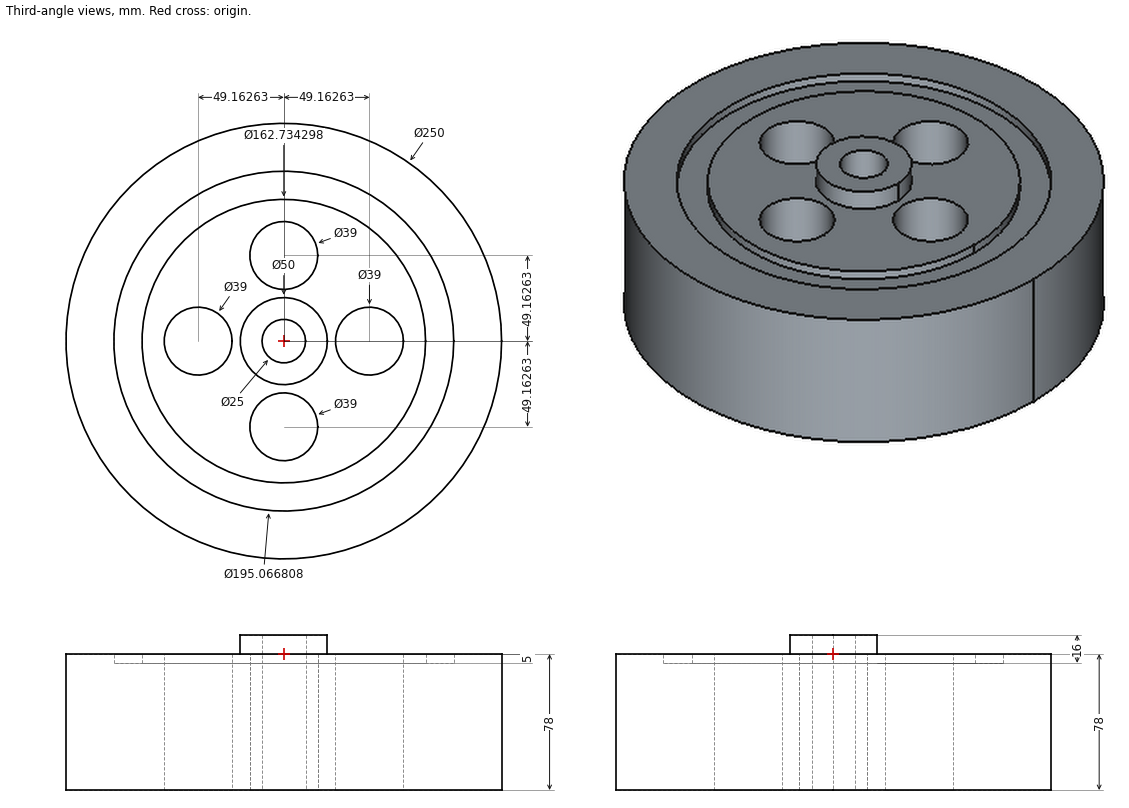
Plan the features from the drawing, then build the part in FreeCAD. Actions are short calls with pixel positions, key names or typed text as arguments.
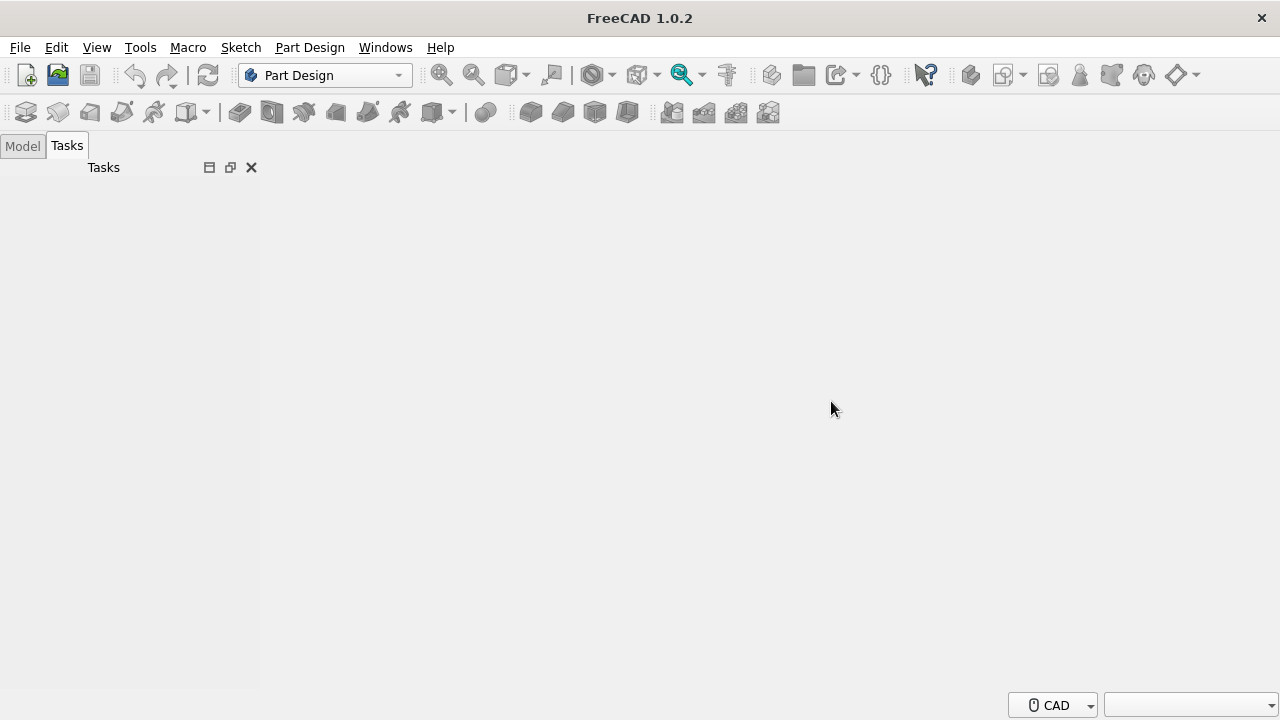
click(26, 76)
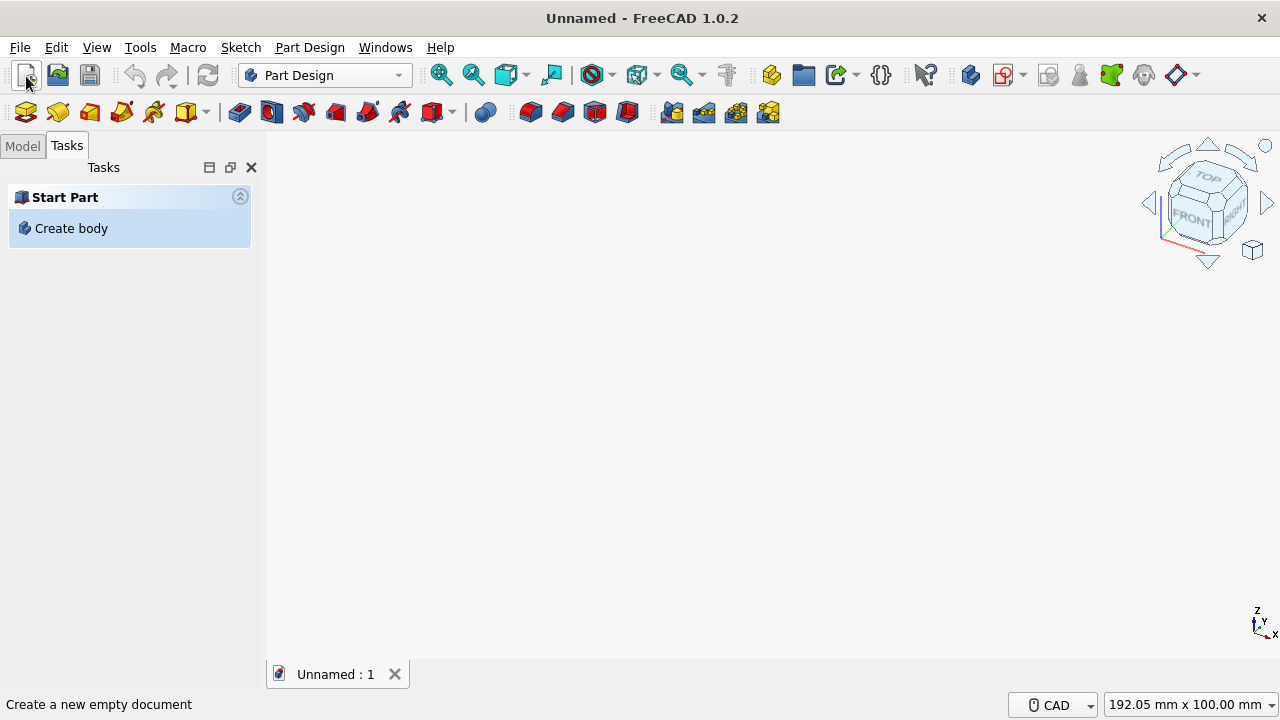
click(1004, 76)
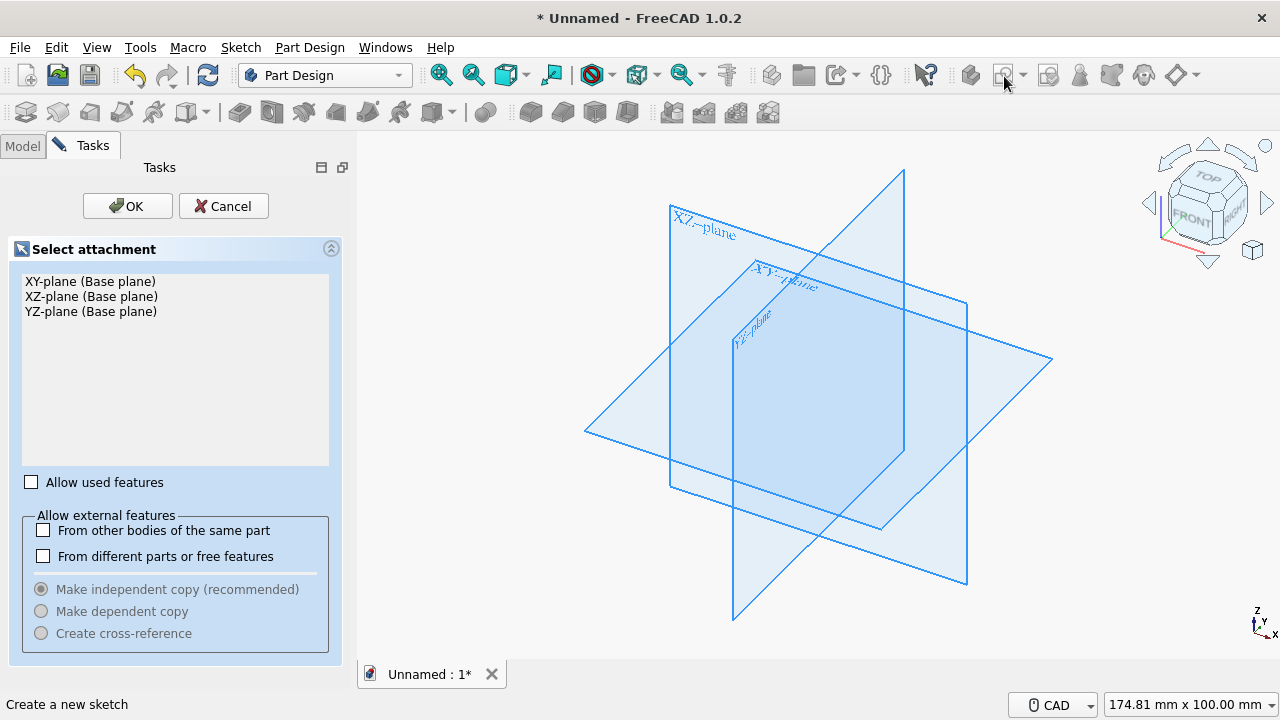
click(82, 282)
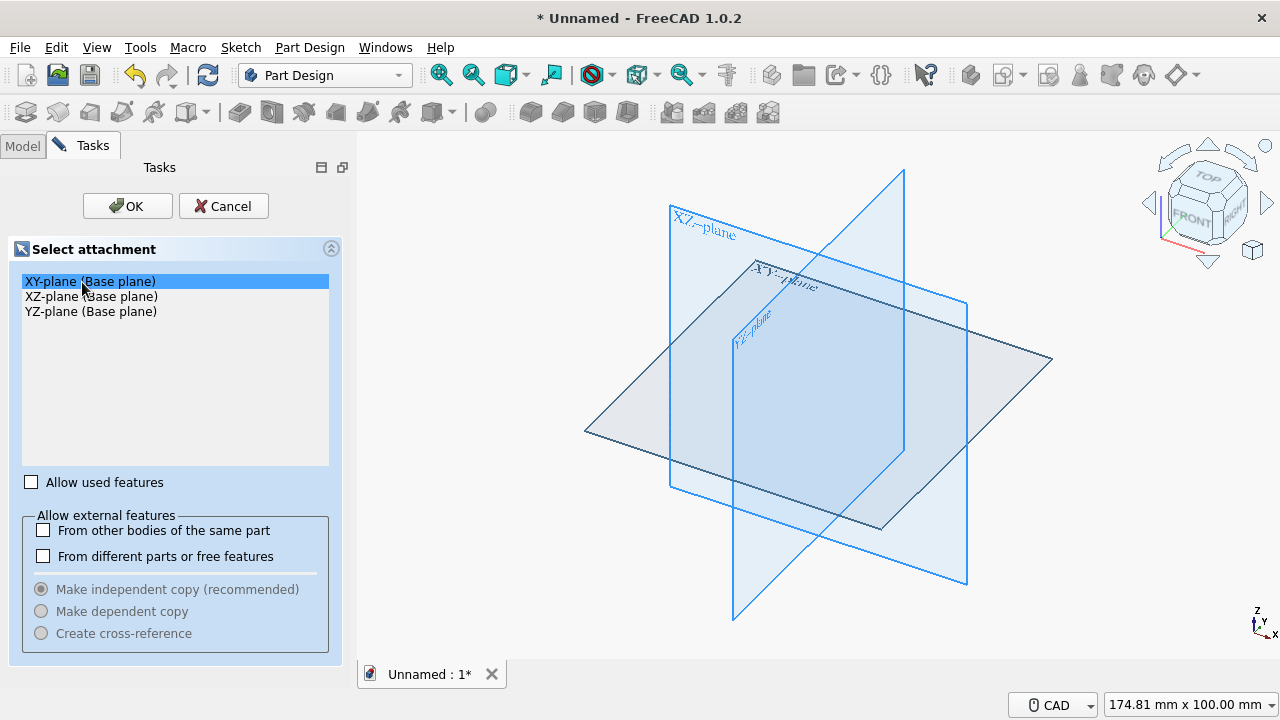
click(128, 206)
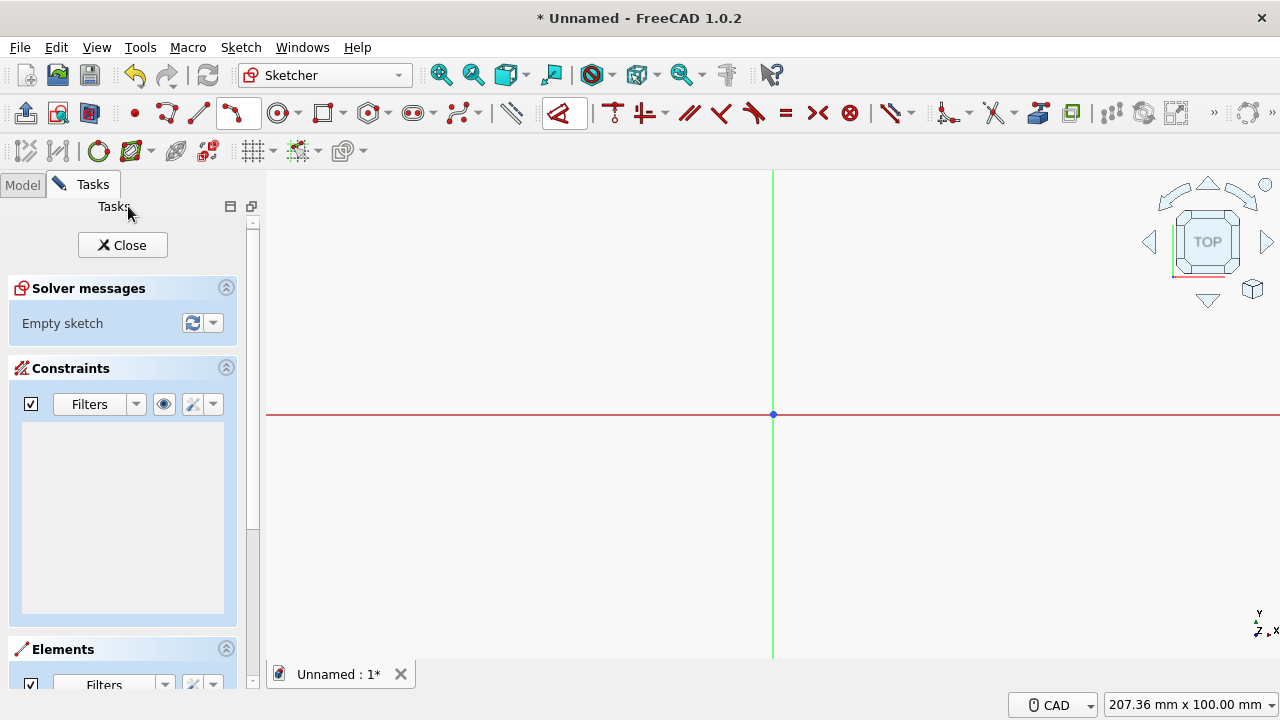
scroll(682, 415, down, 7)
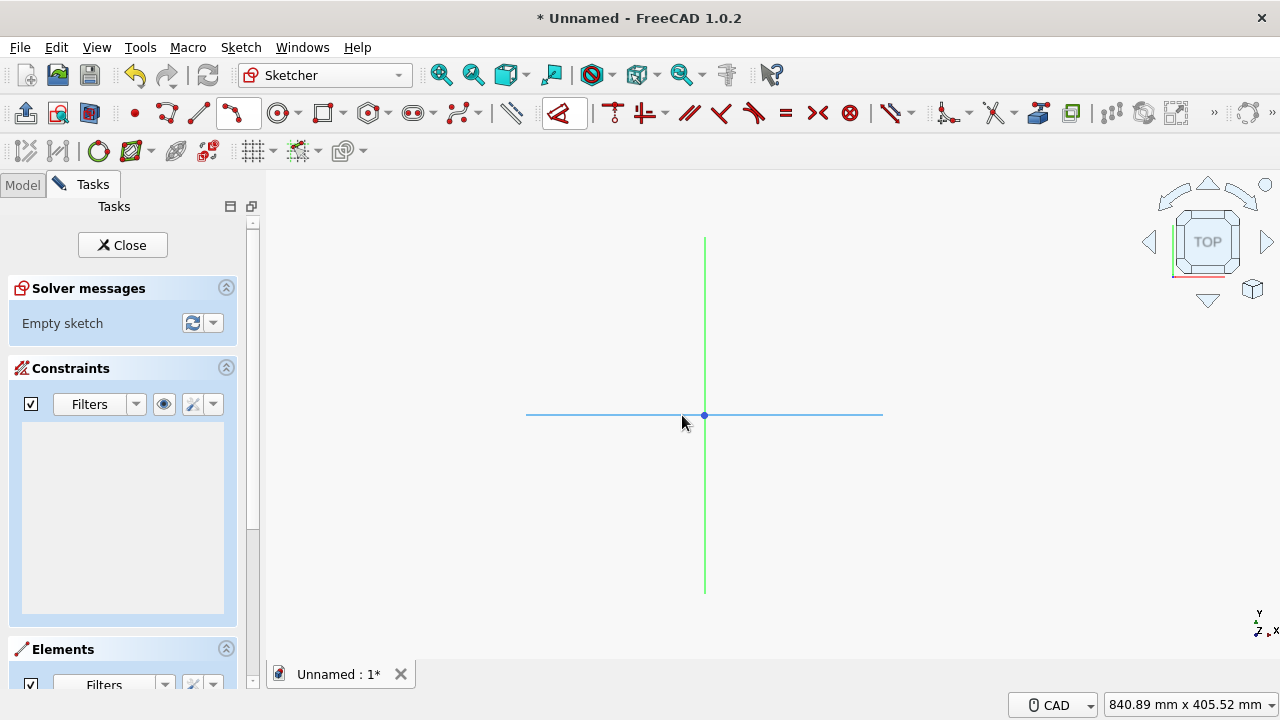
click(278, 114)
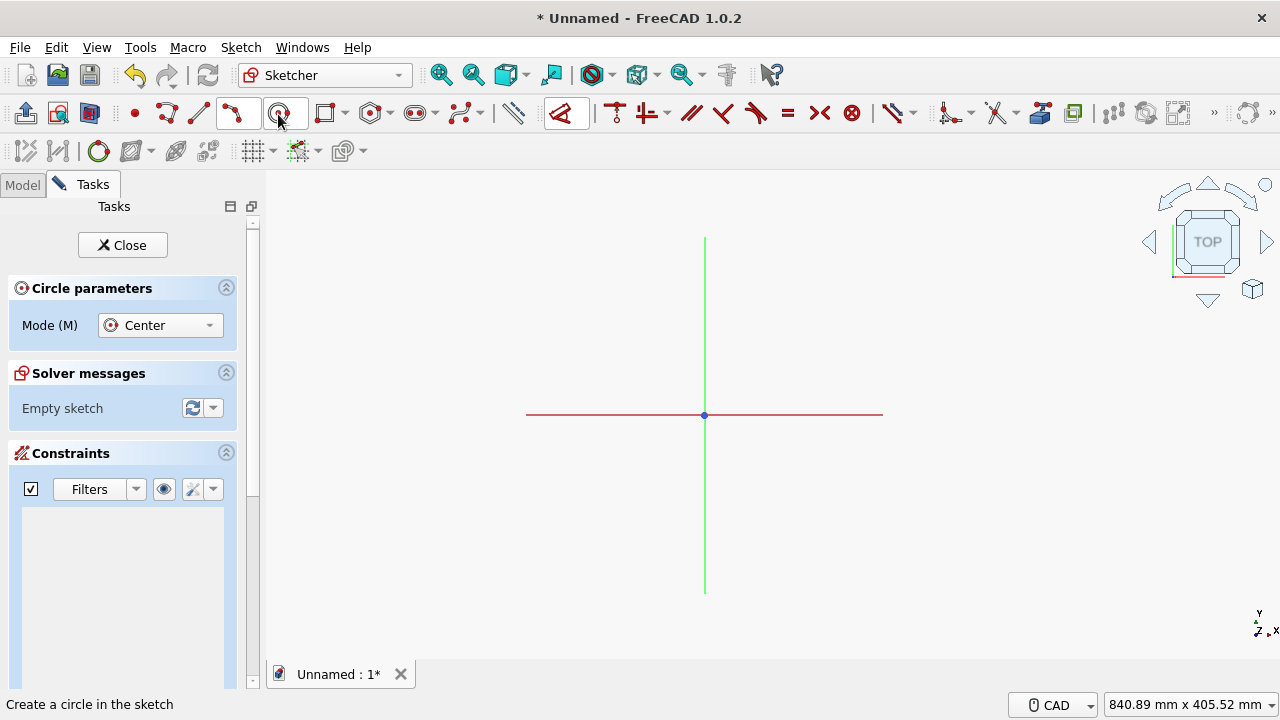
click(705, 415)
move(811, 309)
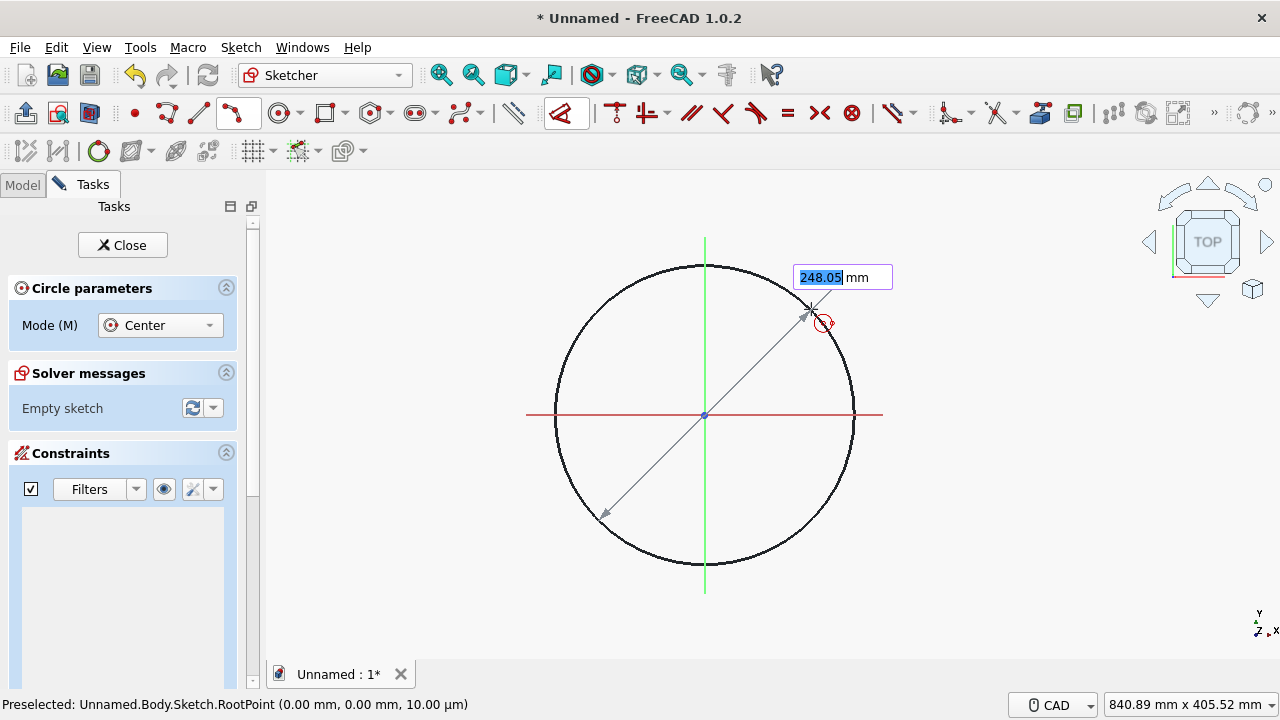
text(250)
key(Return)
key(Escape)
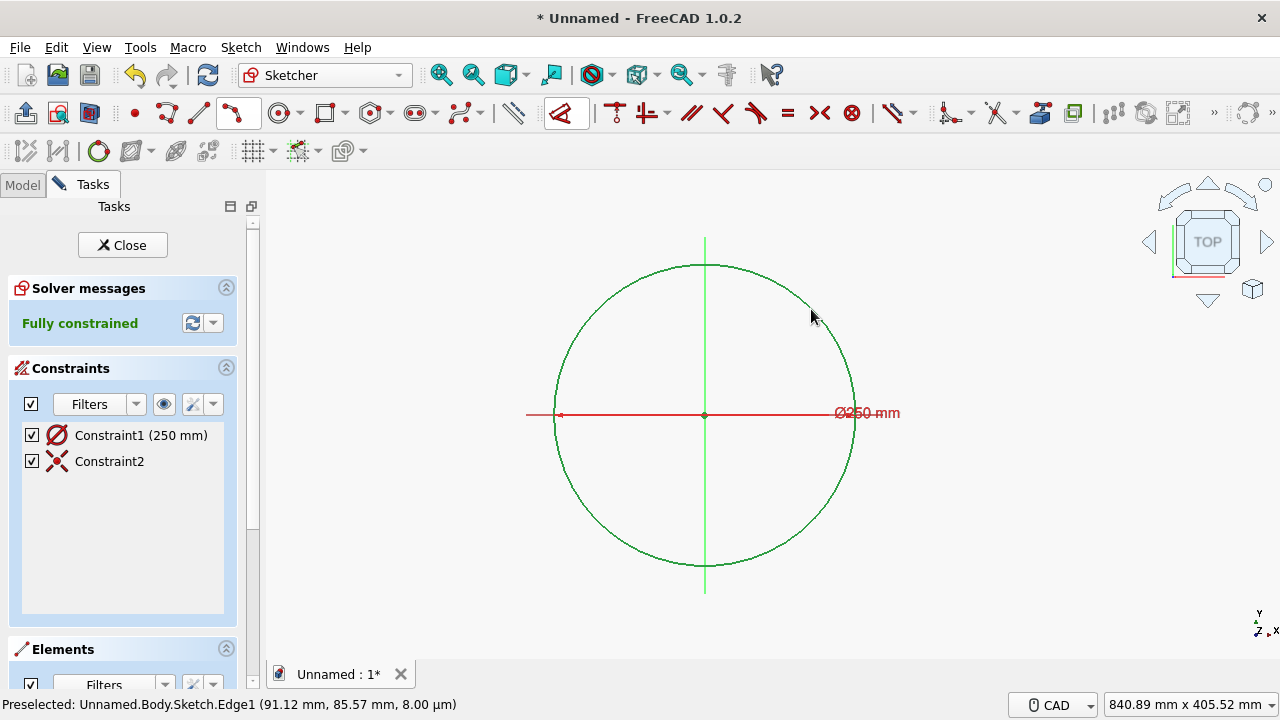
click(123, 245)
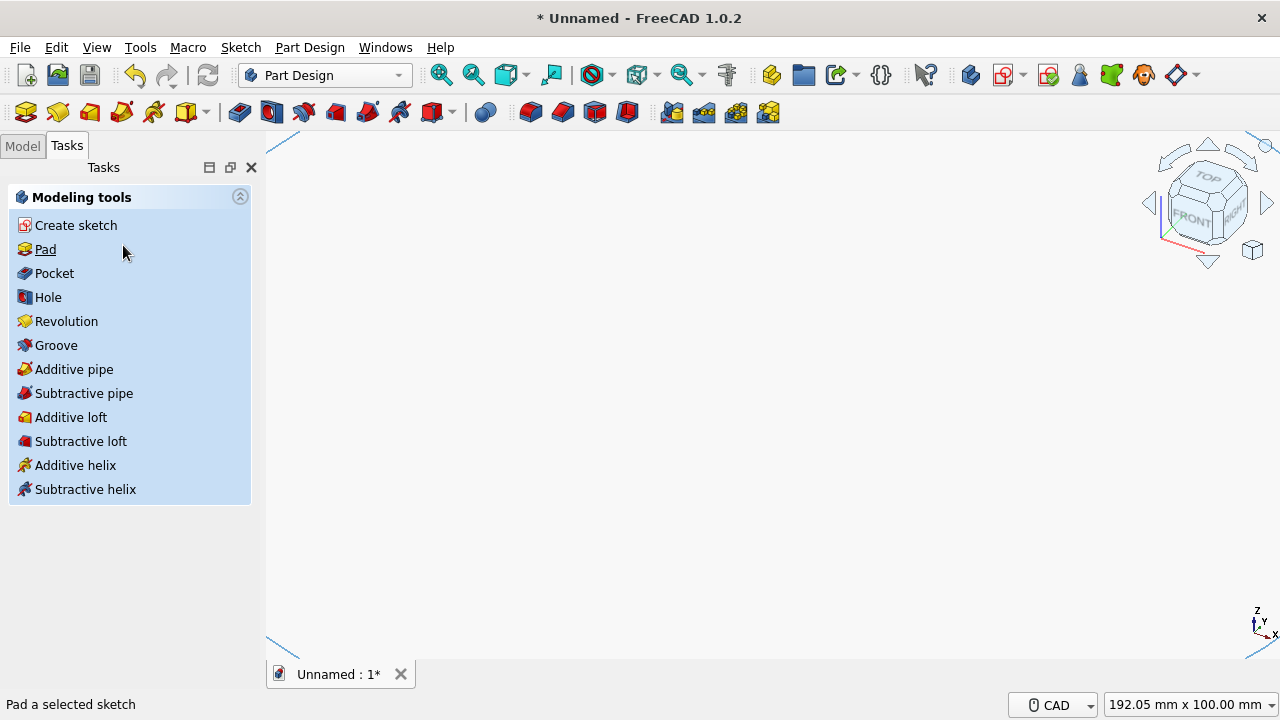
click(26, 112)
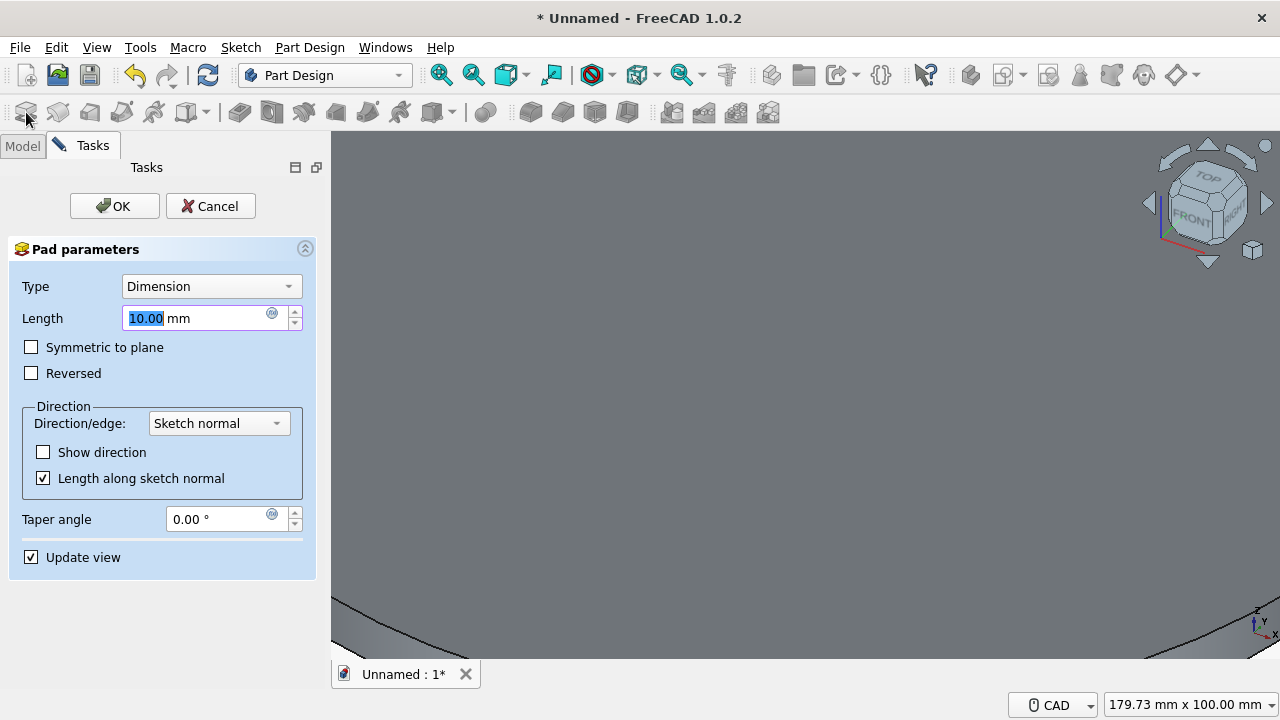
text(78)
key(Tab)